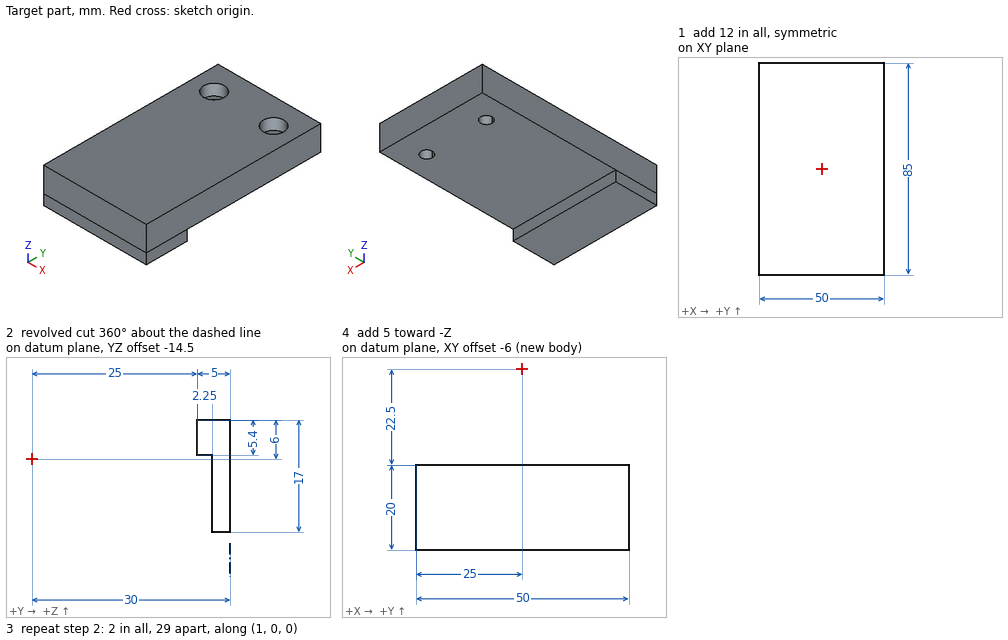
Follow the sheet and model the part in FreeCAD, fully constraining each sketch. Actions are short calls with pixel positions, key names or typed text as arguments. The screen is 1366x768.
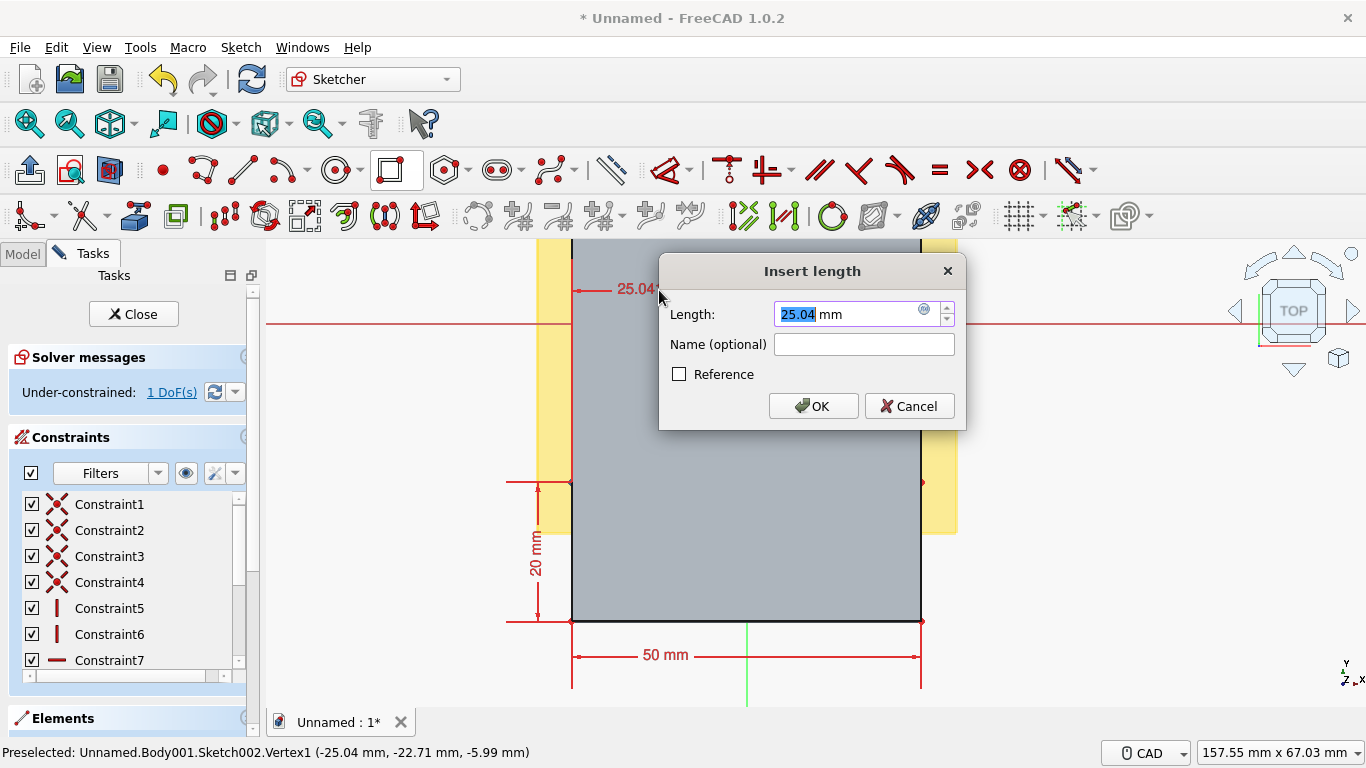
text(25)
key(Return)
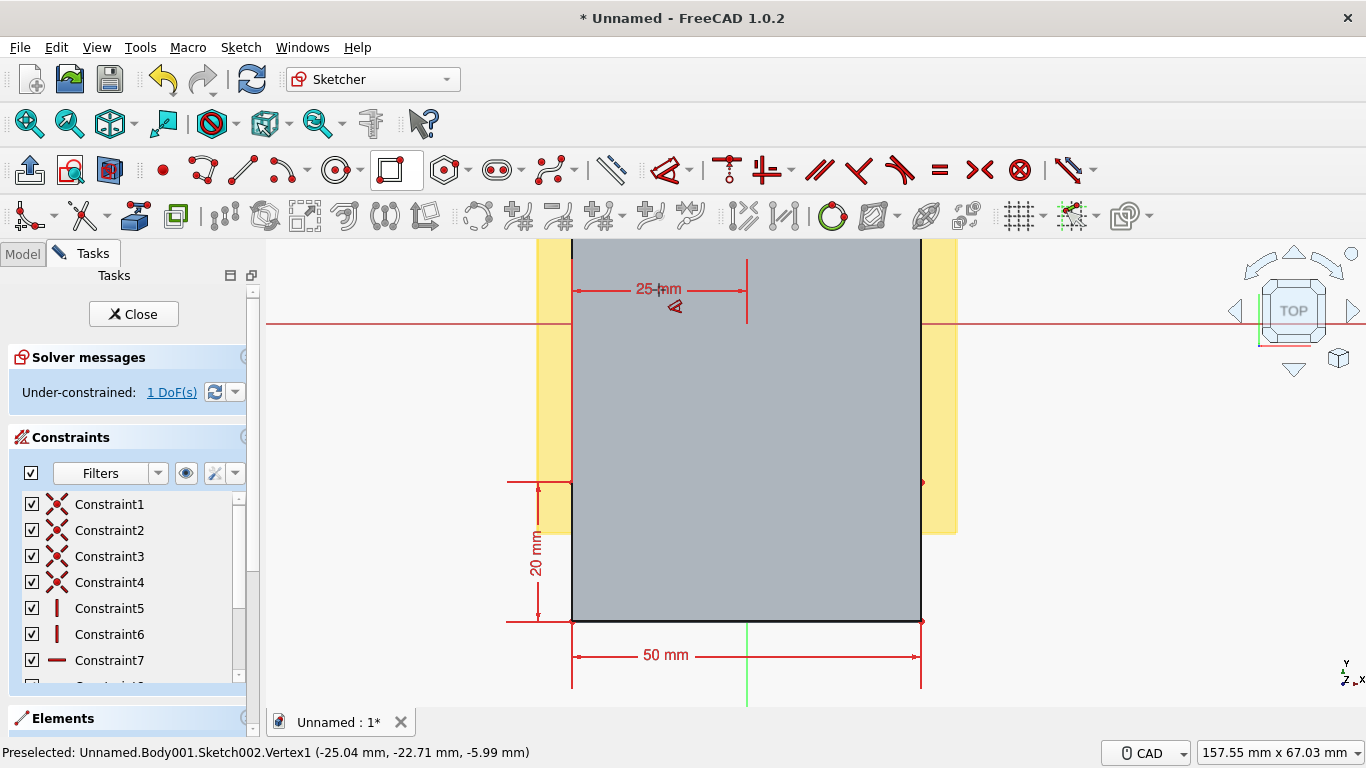
click(572, 482)
click(538, 403)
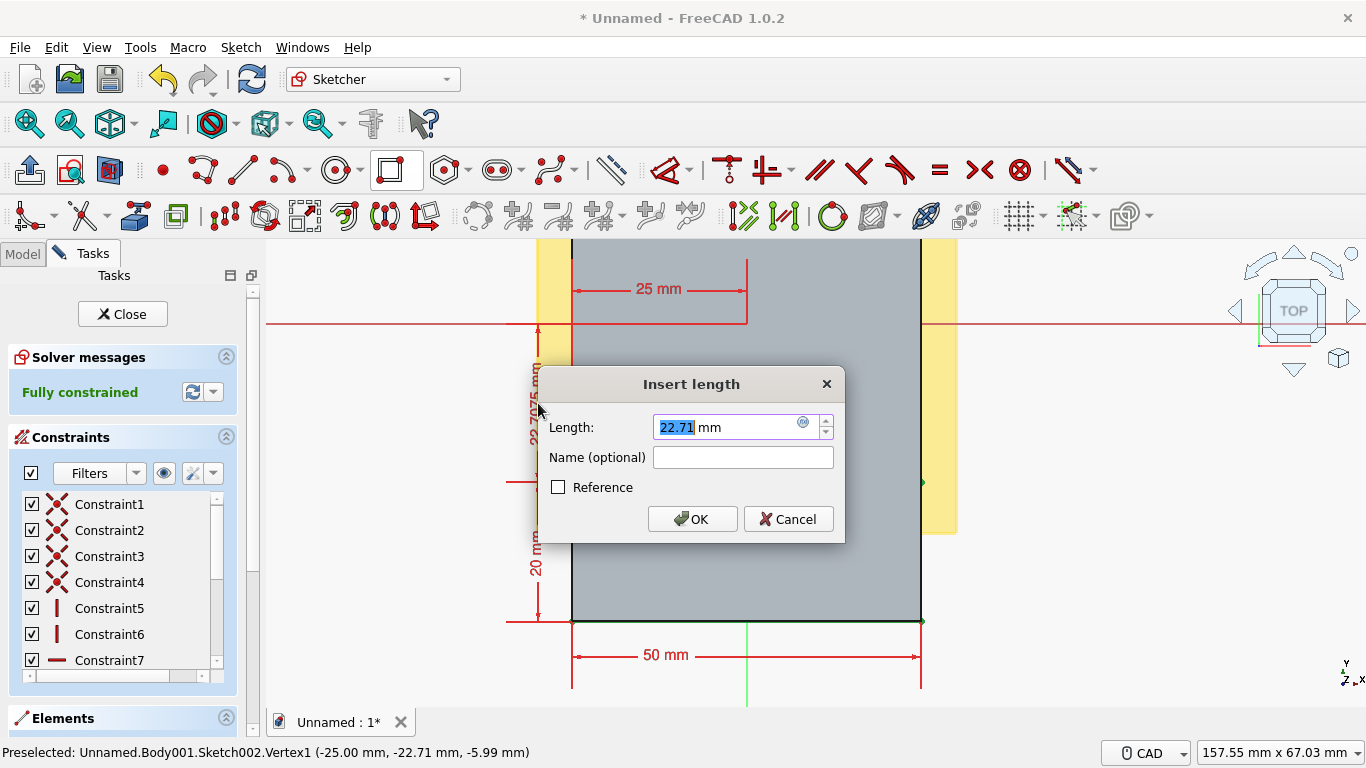
text(22.5)
key(Return)
key(Escape)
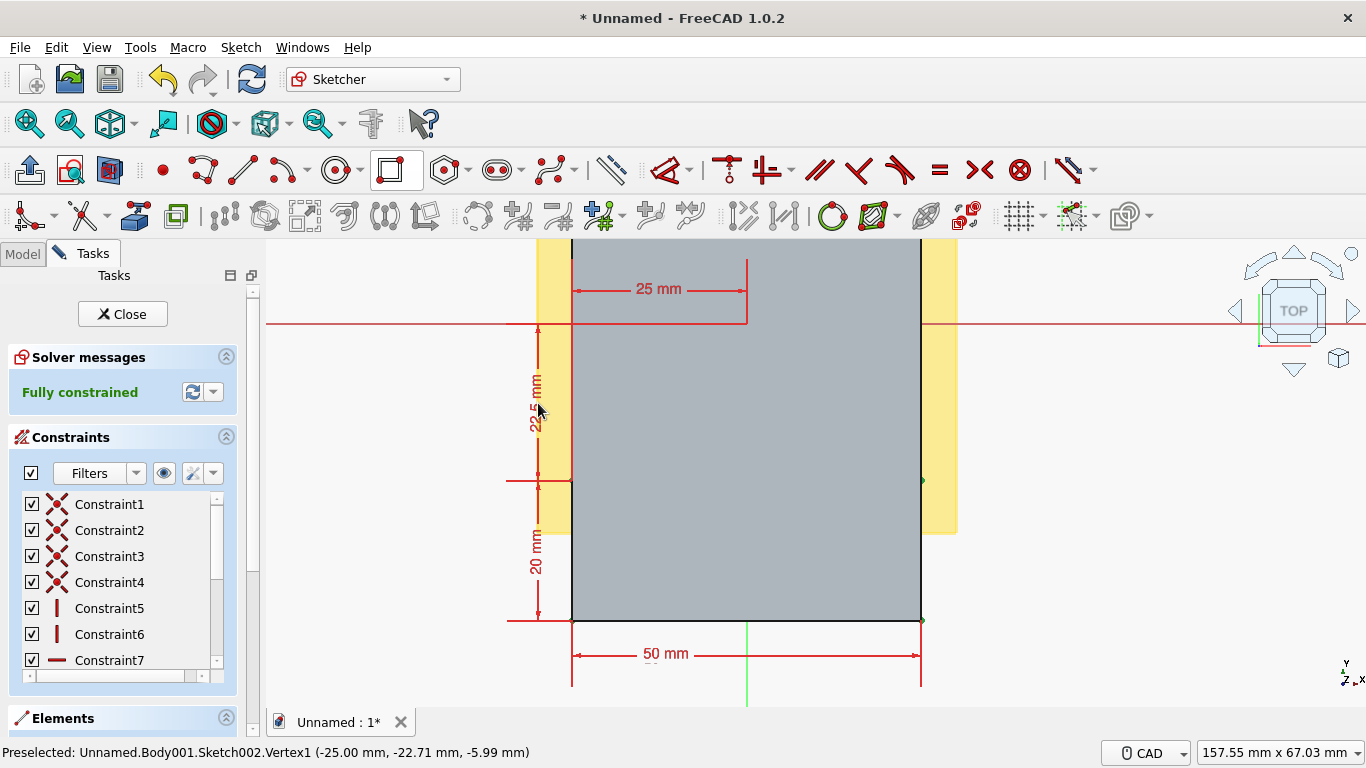
click(123, 314)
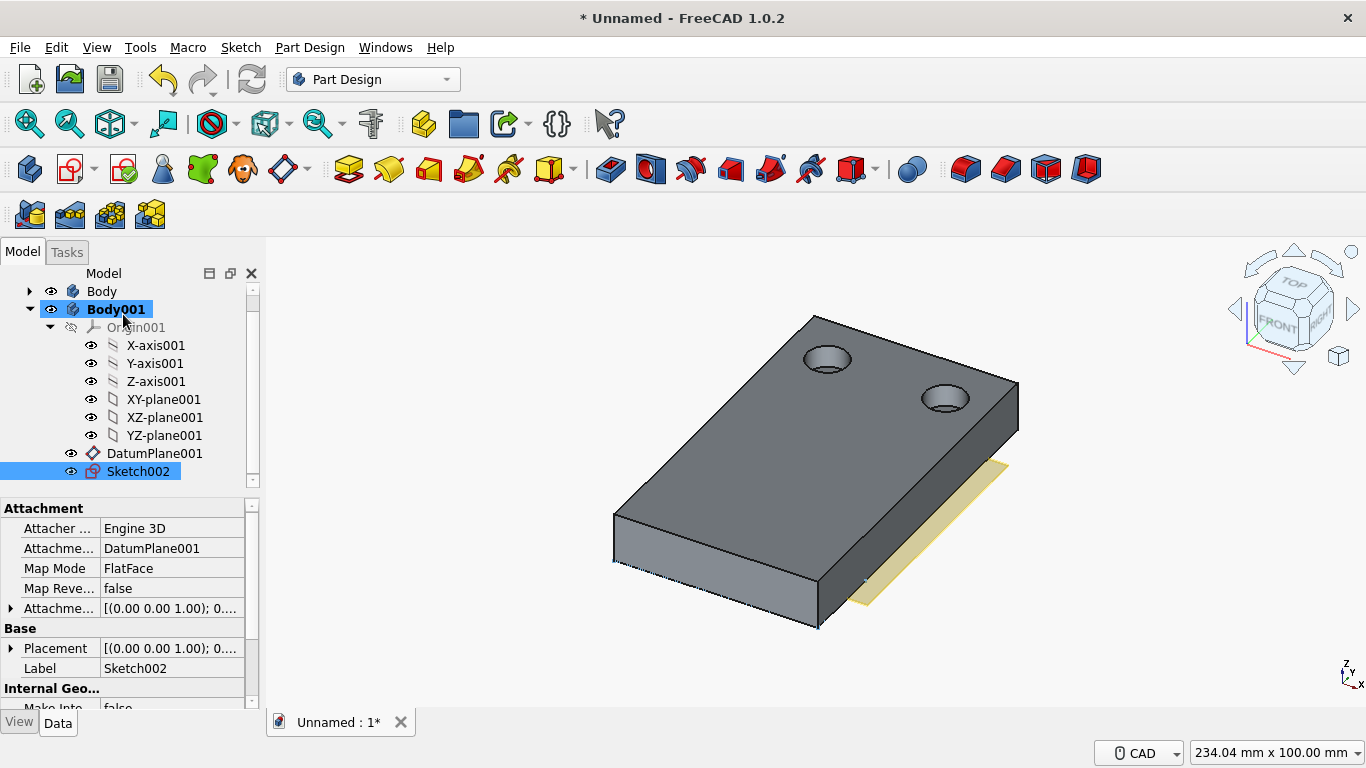
click(350, 170)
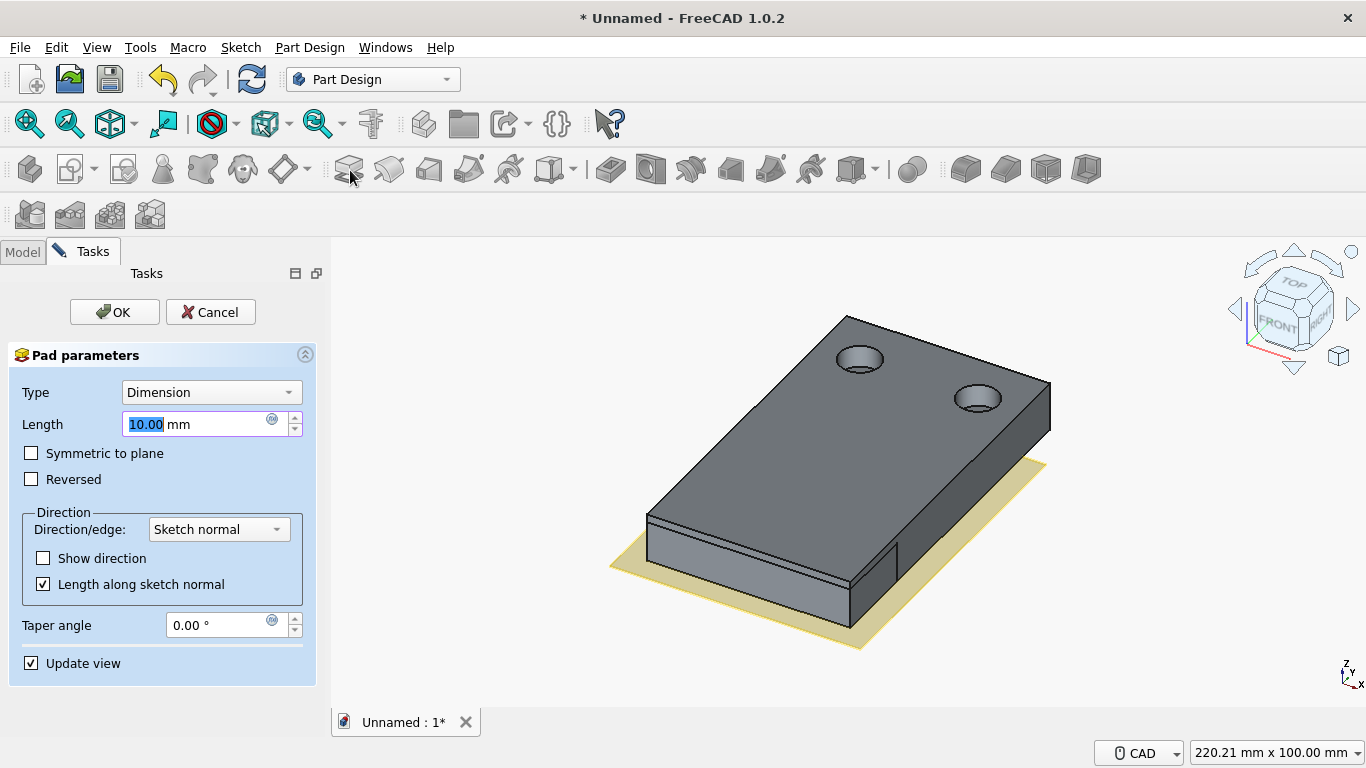
text(5)
key(Tab)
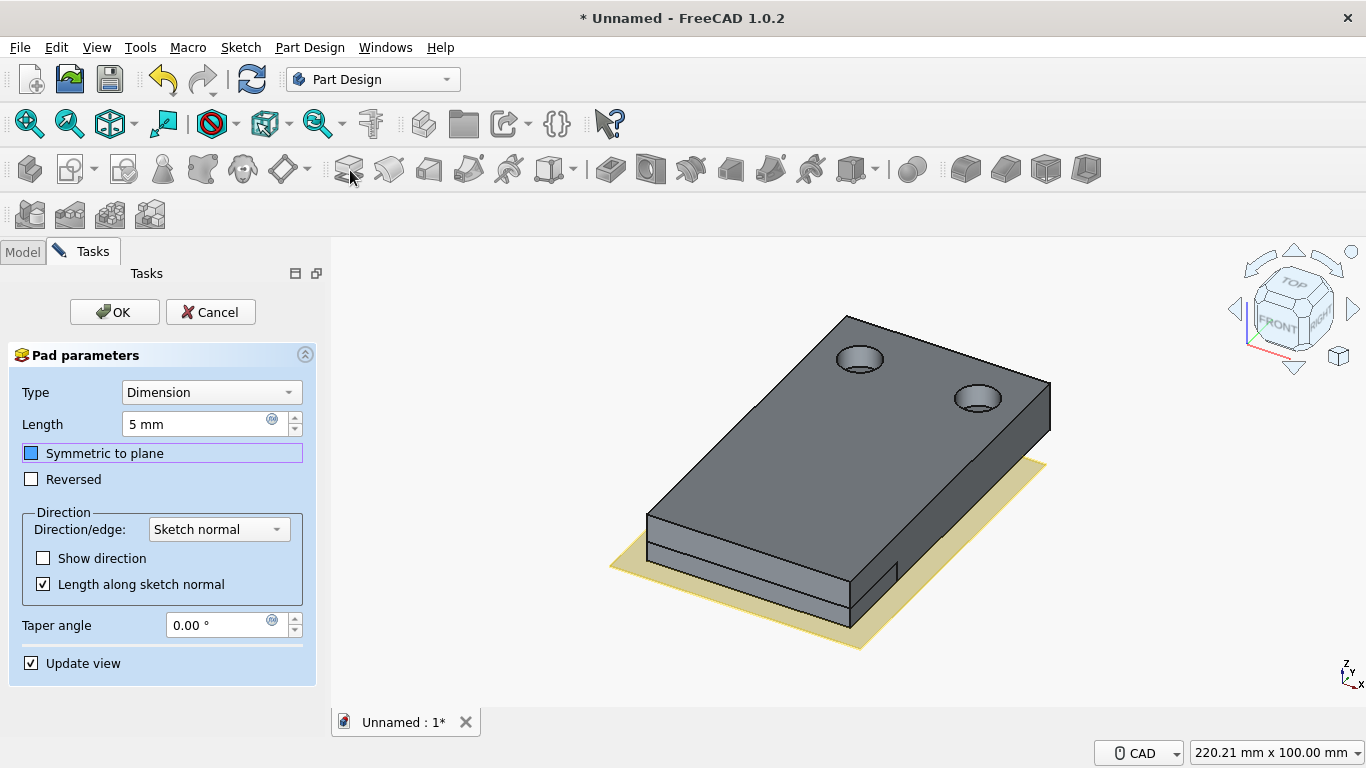
click(30, 479)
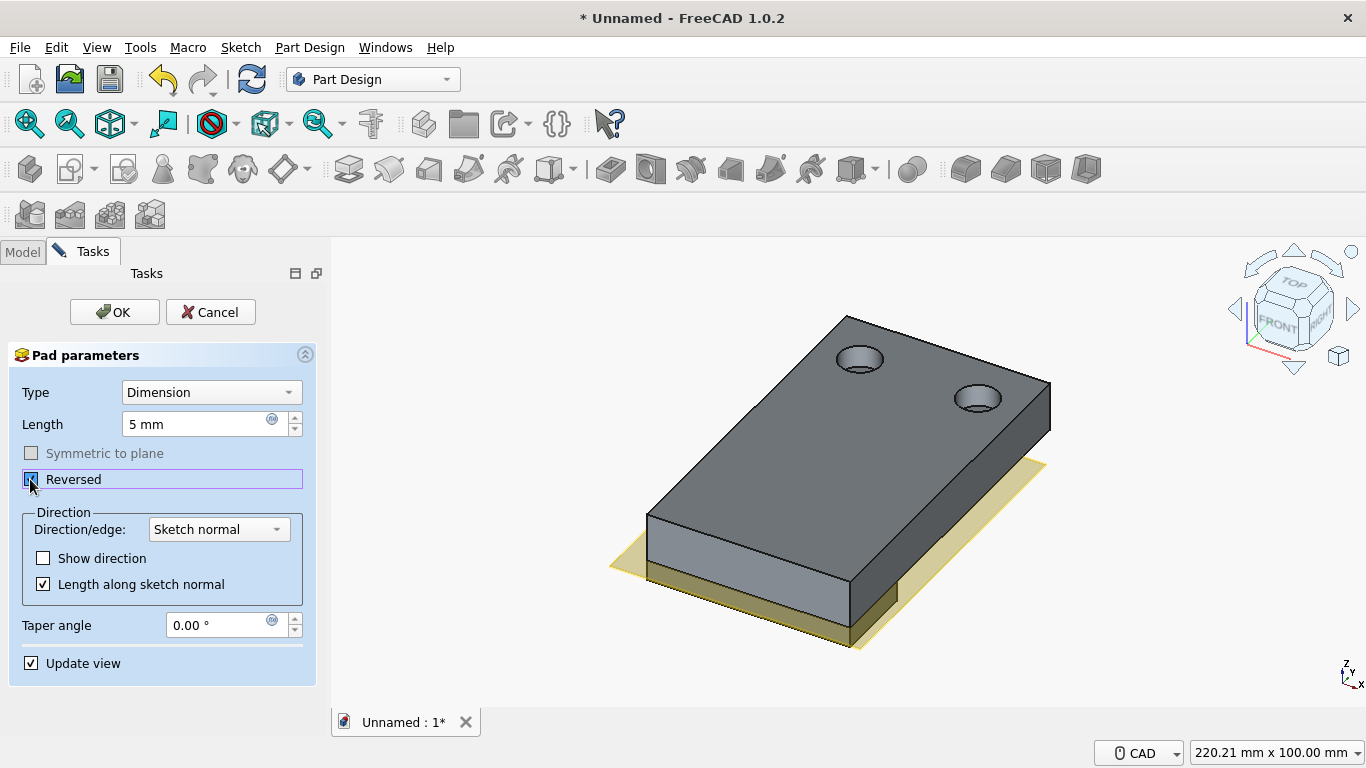
click(115, 312)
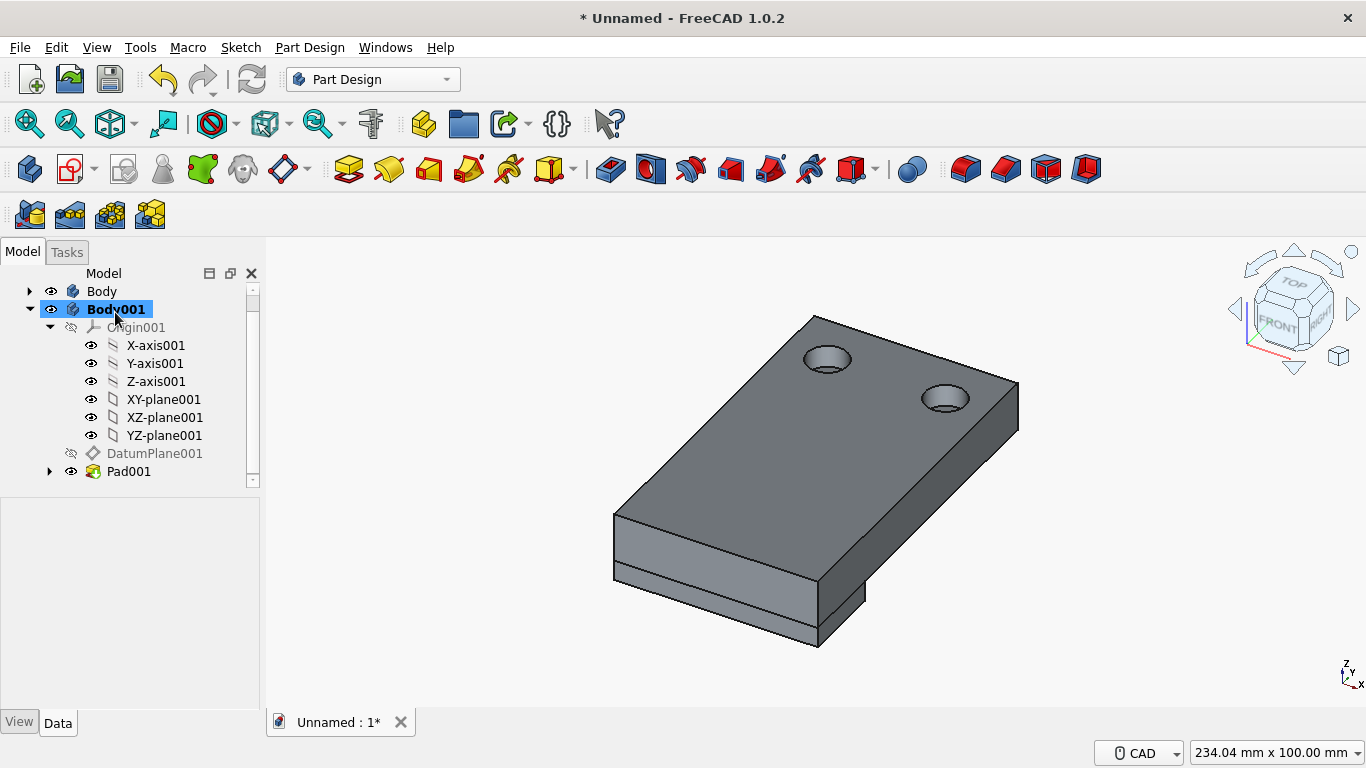
key(0)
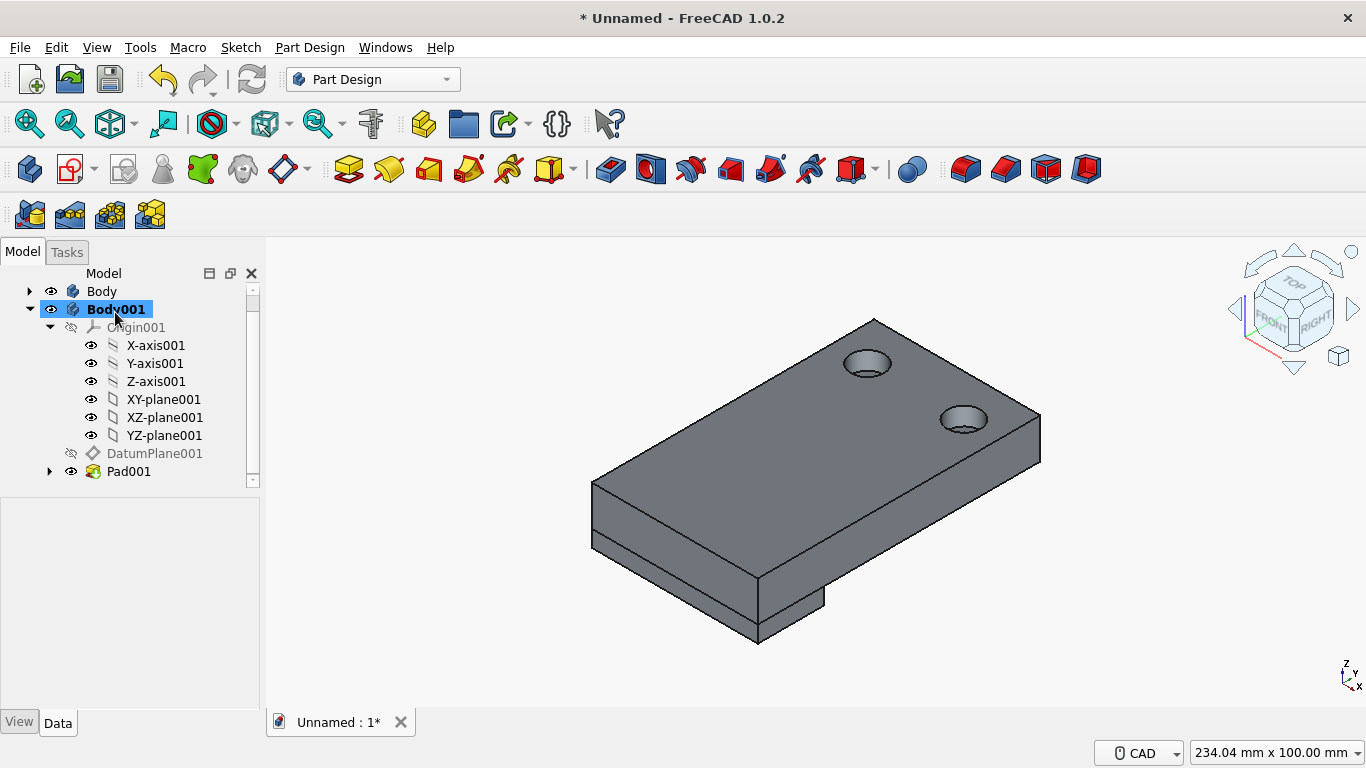
key(v)
key(f)